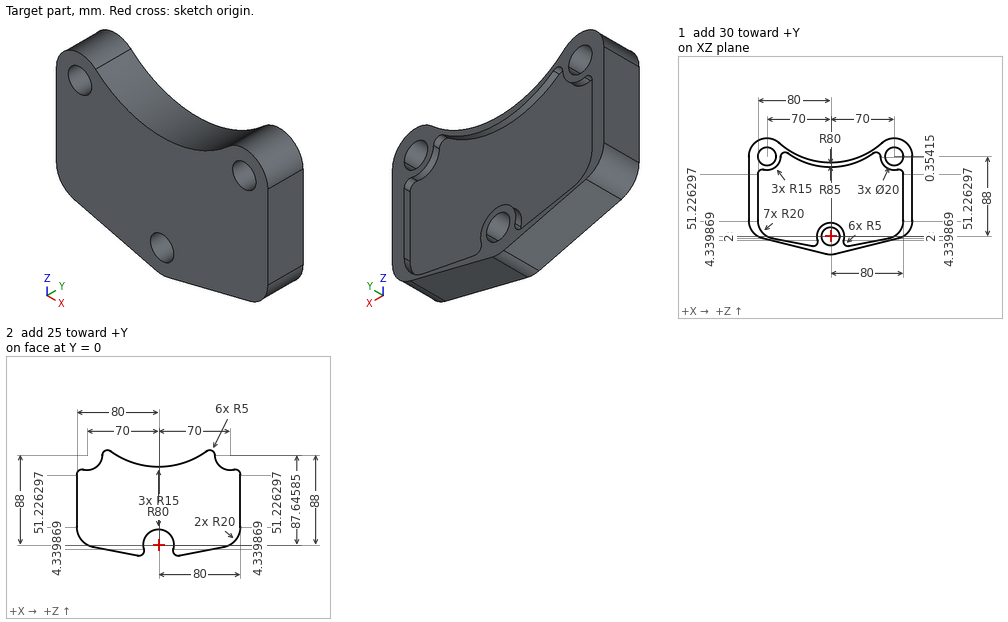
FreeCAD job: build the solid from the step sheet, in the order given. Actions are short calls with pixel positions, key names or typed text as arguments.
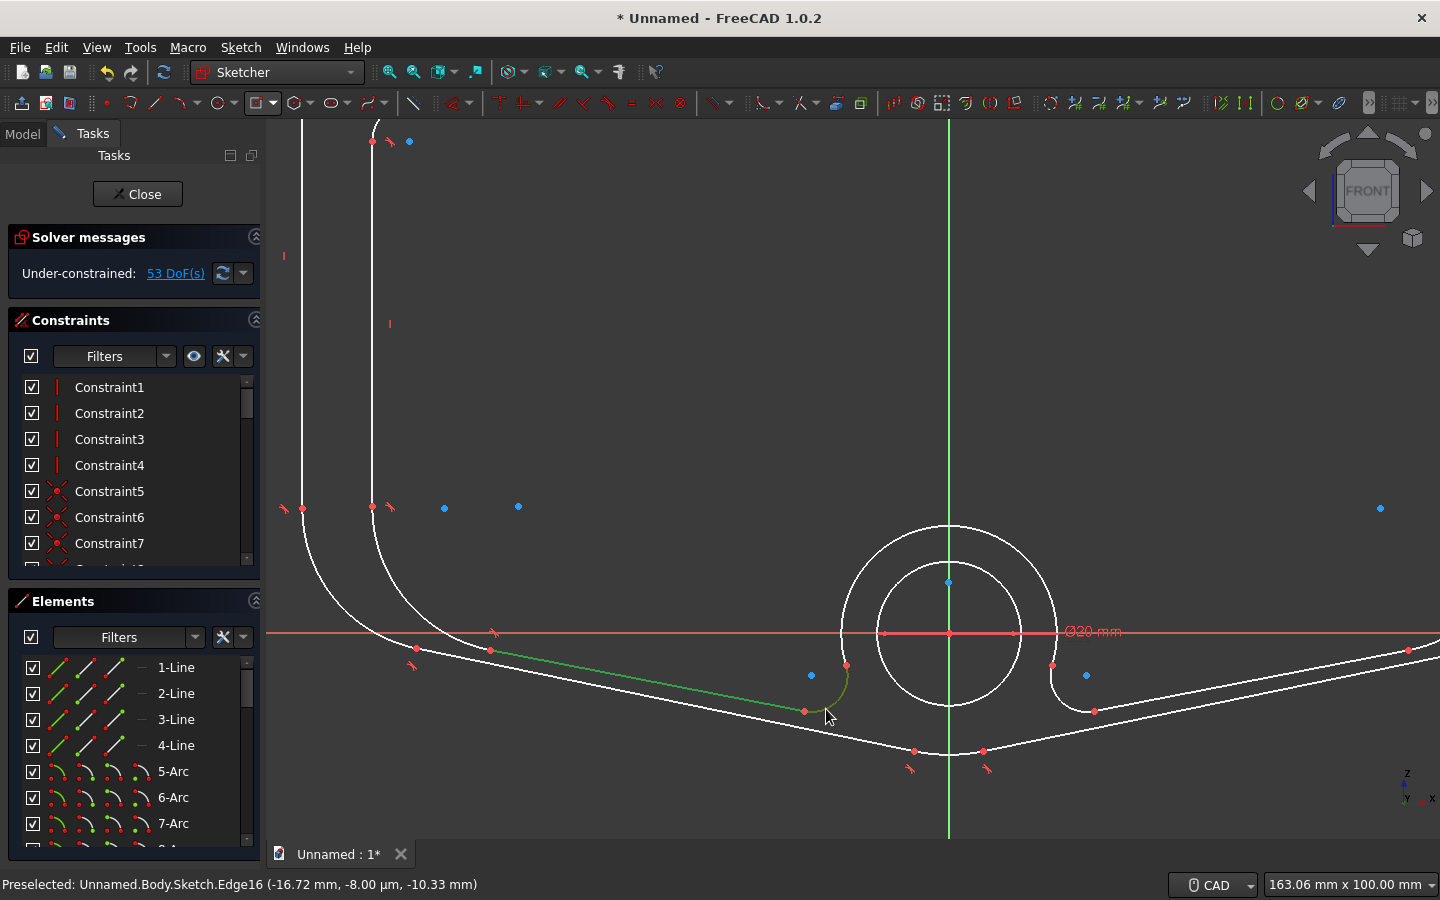
key(t)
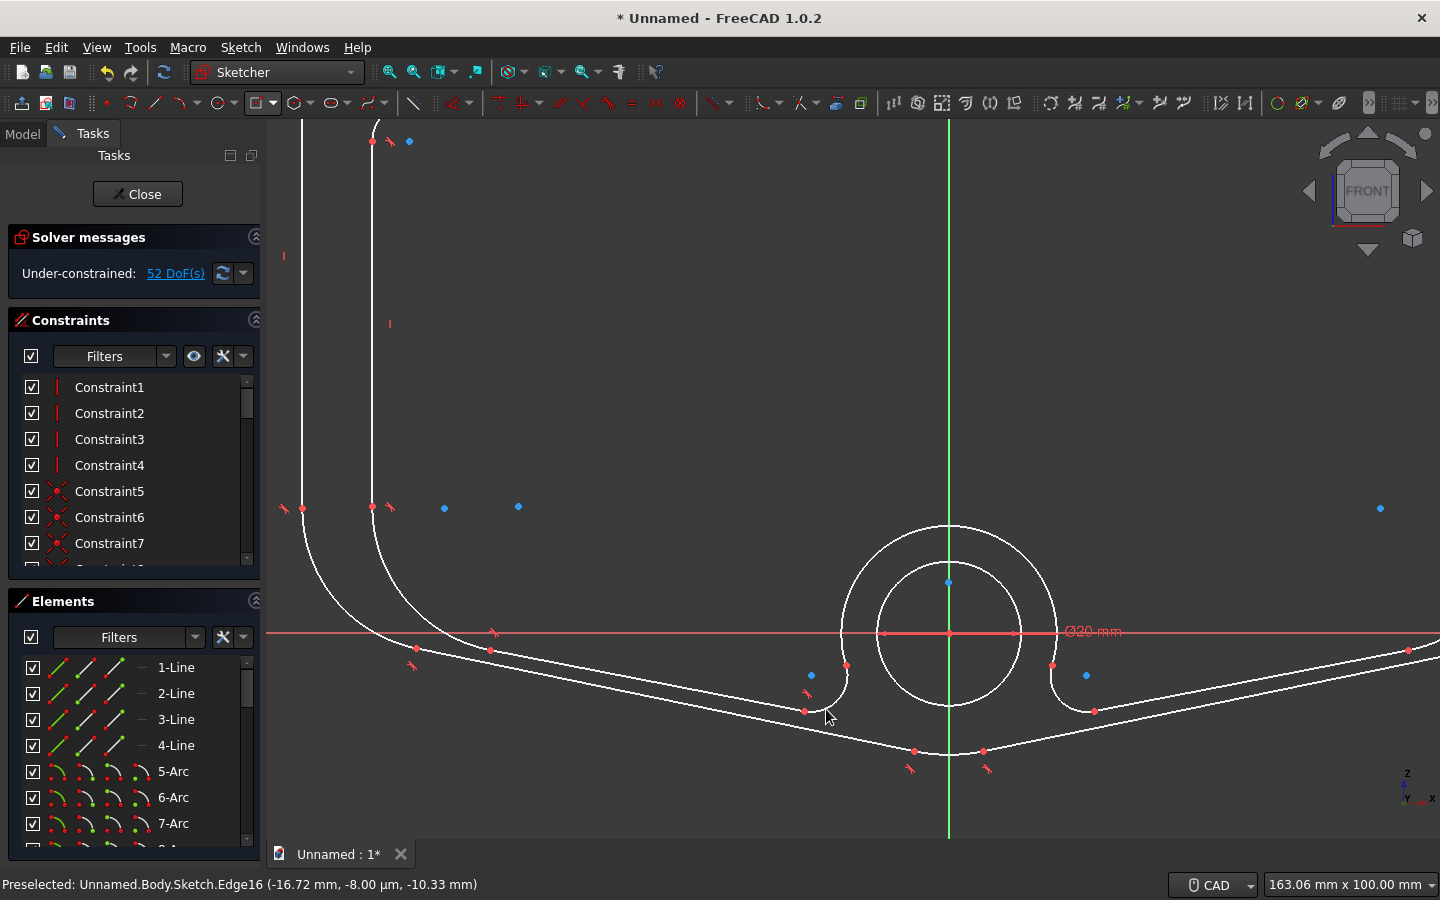
click(1188, 693)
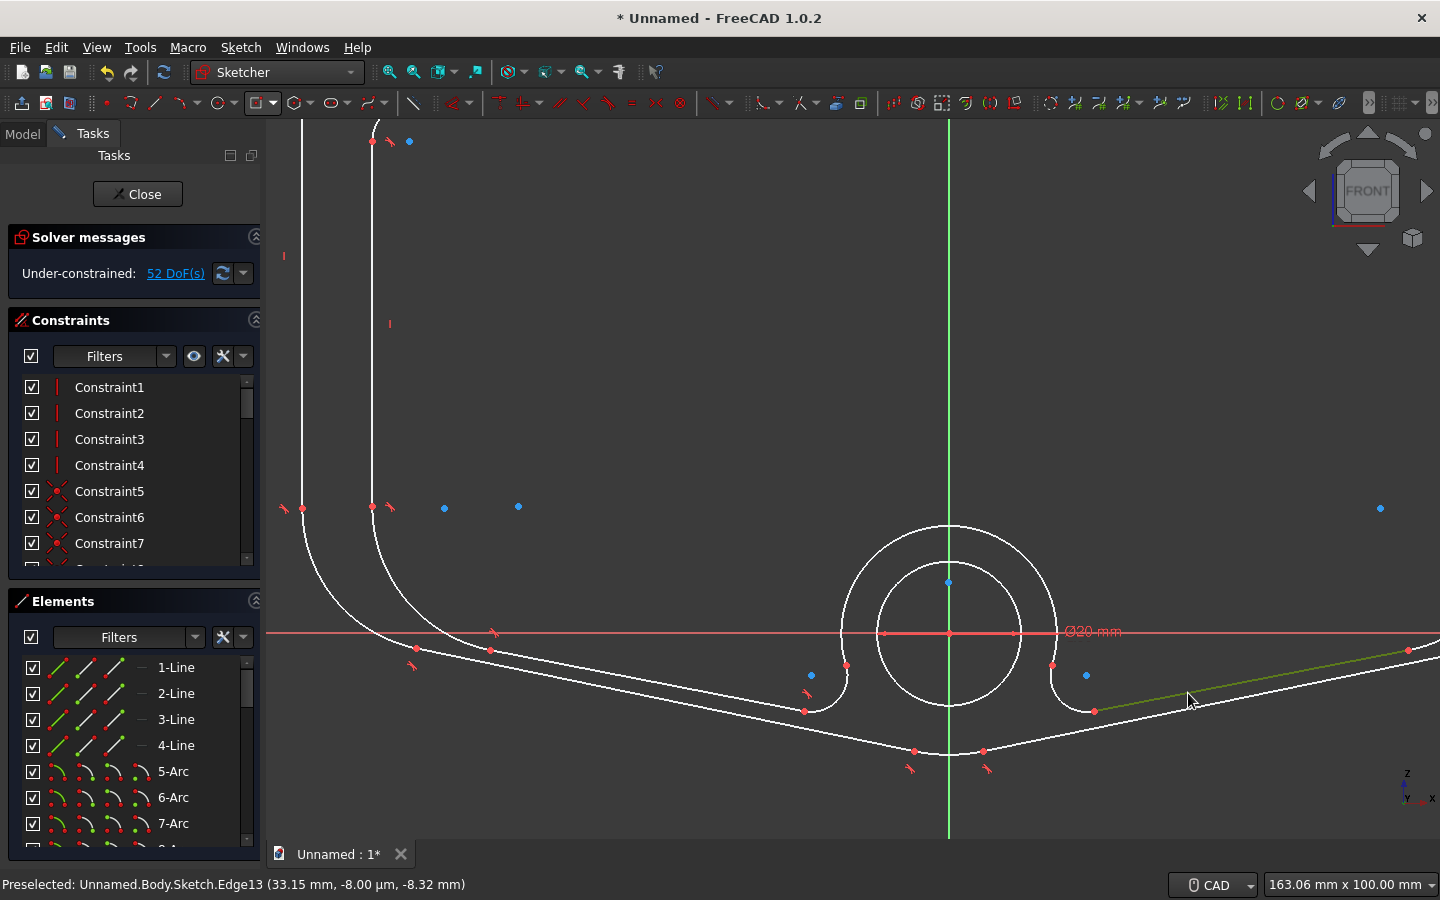
click(1052, 687)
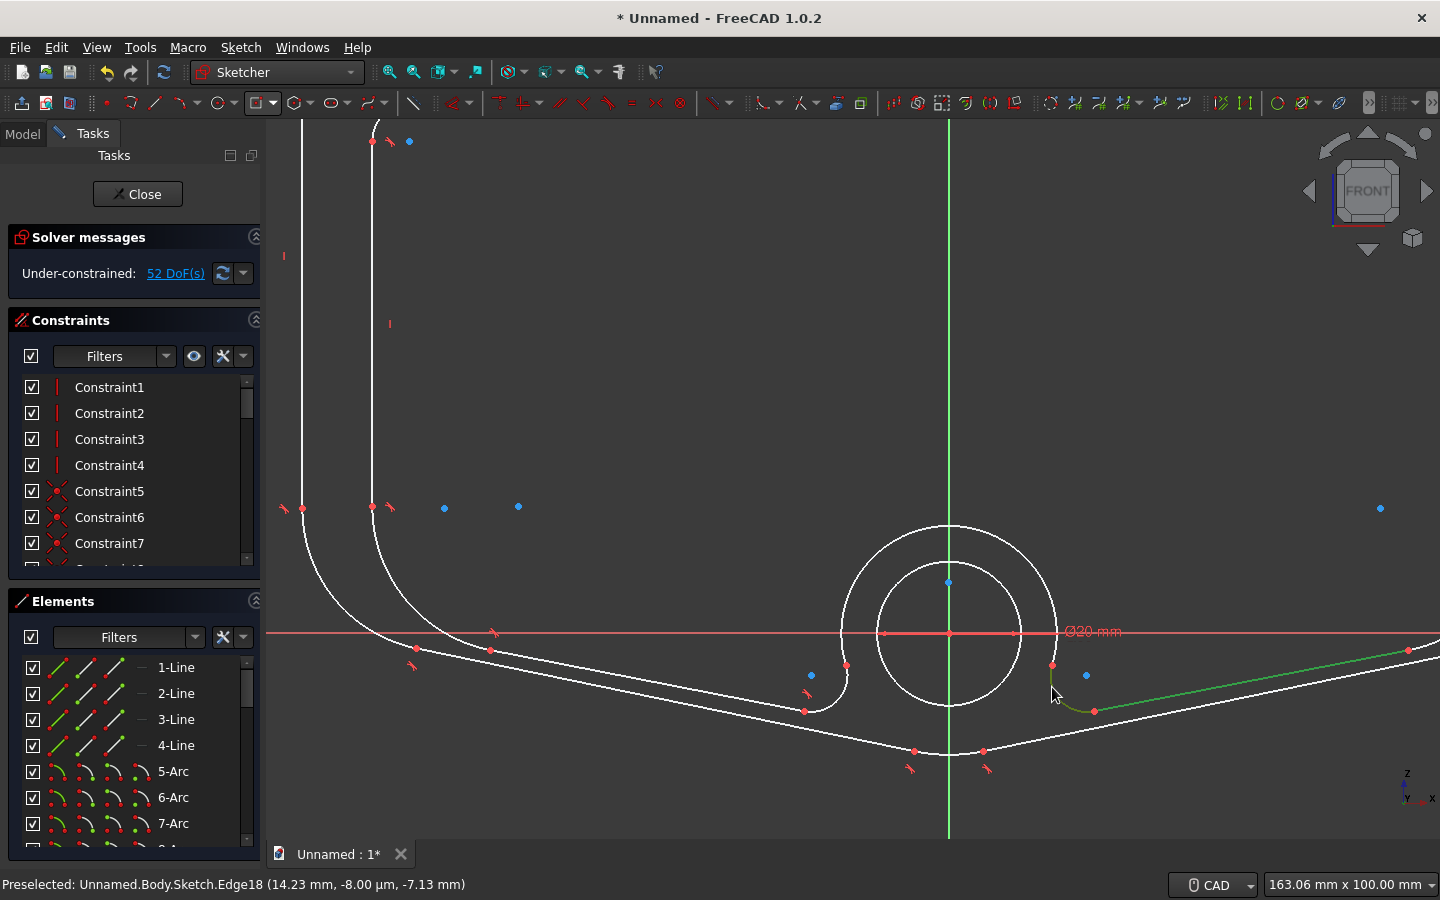
click(608, 104)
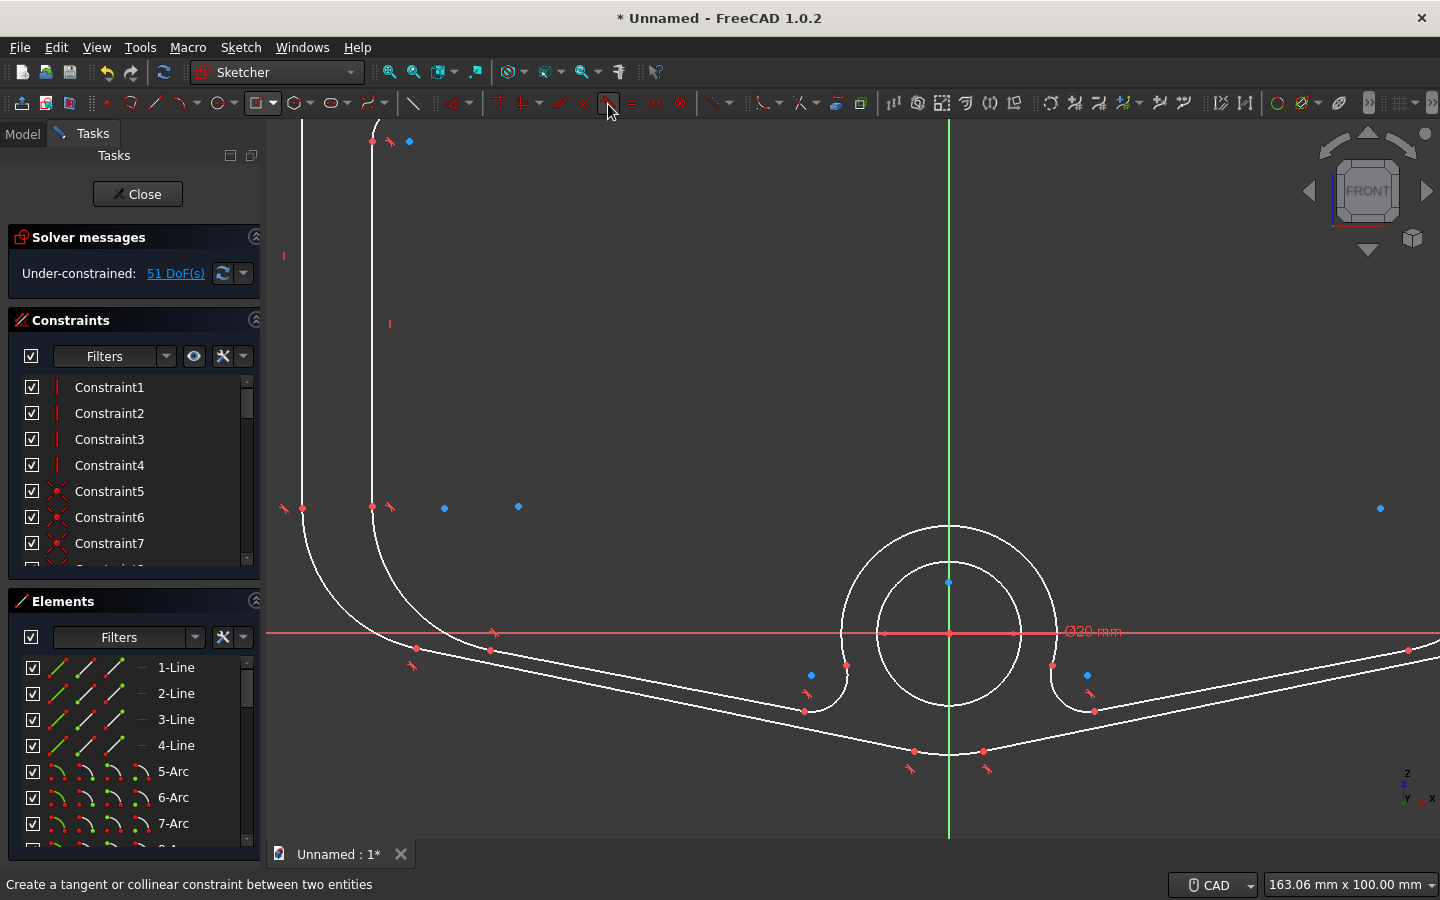
click(1188, 693)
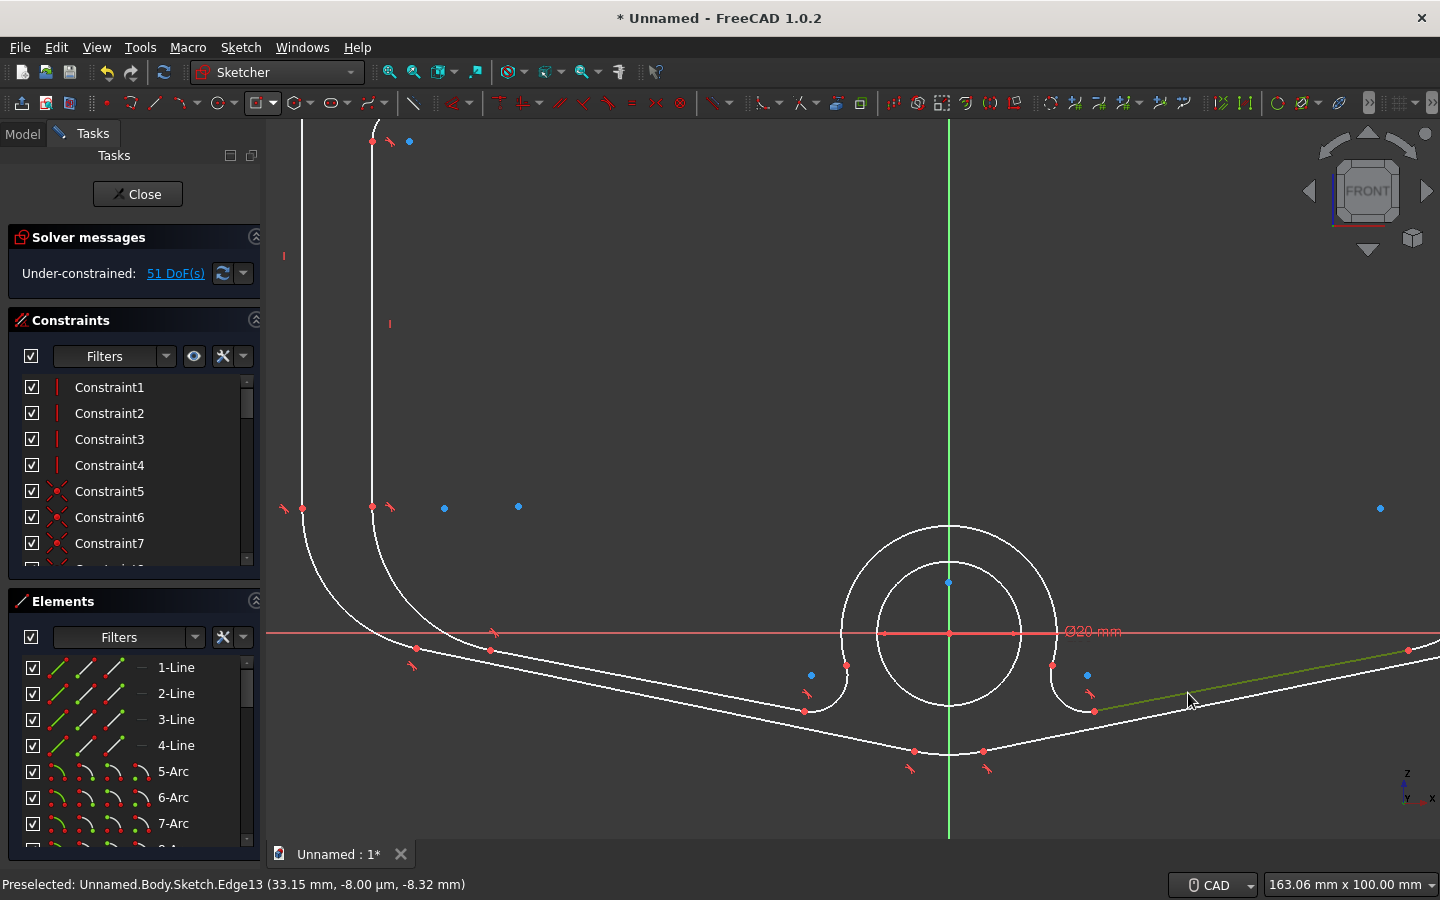
scroll(584, 669, down, 3)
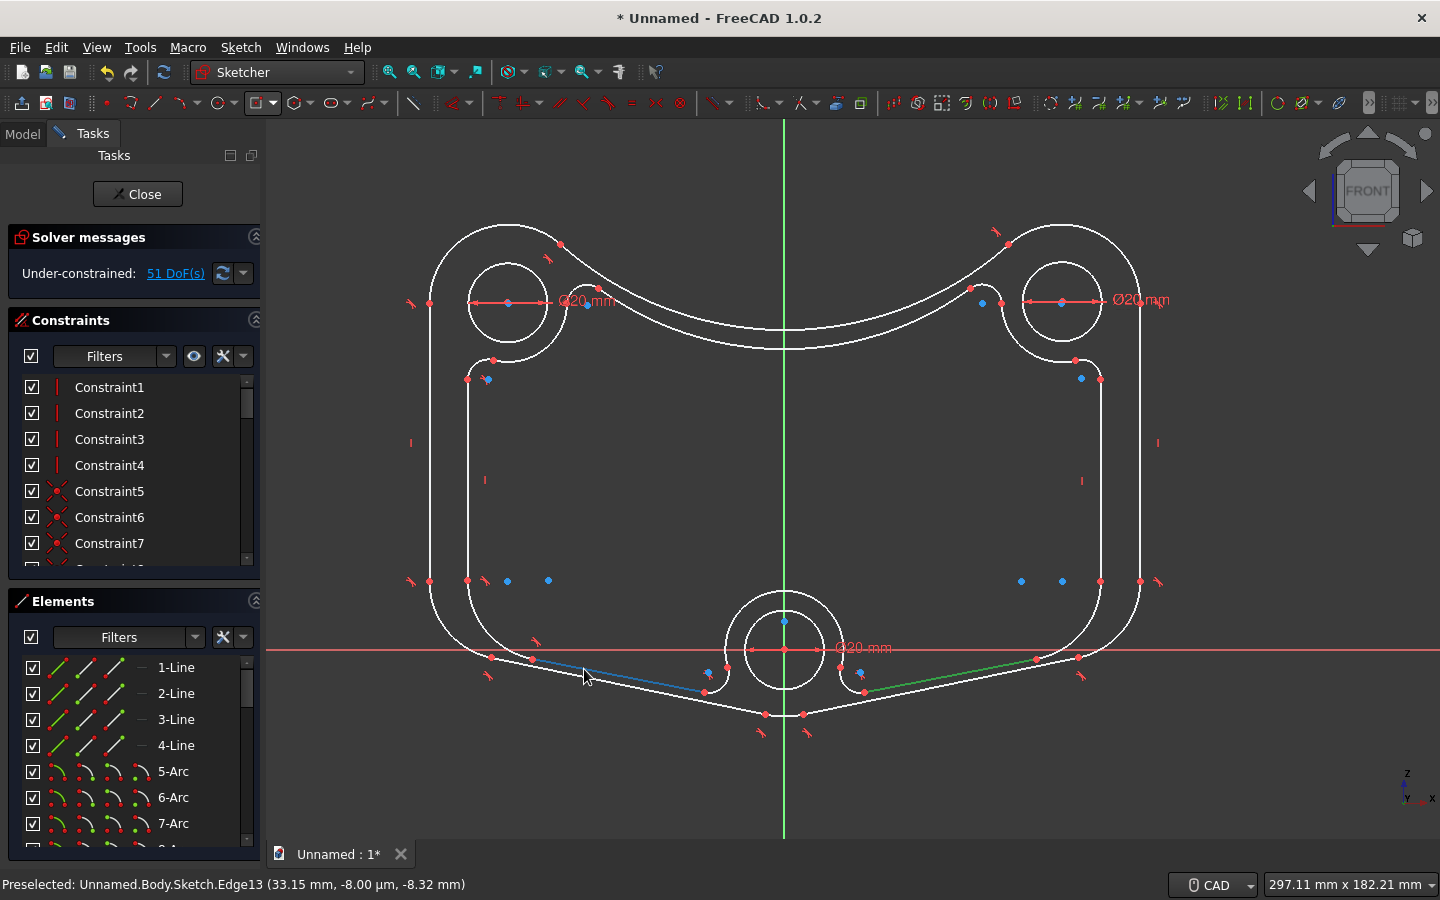
click(1094, 613)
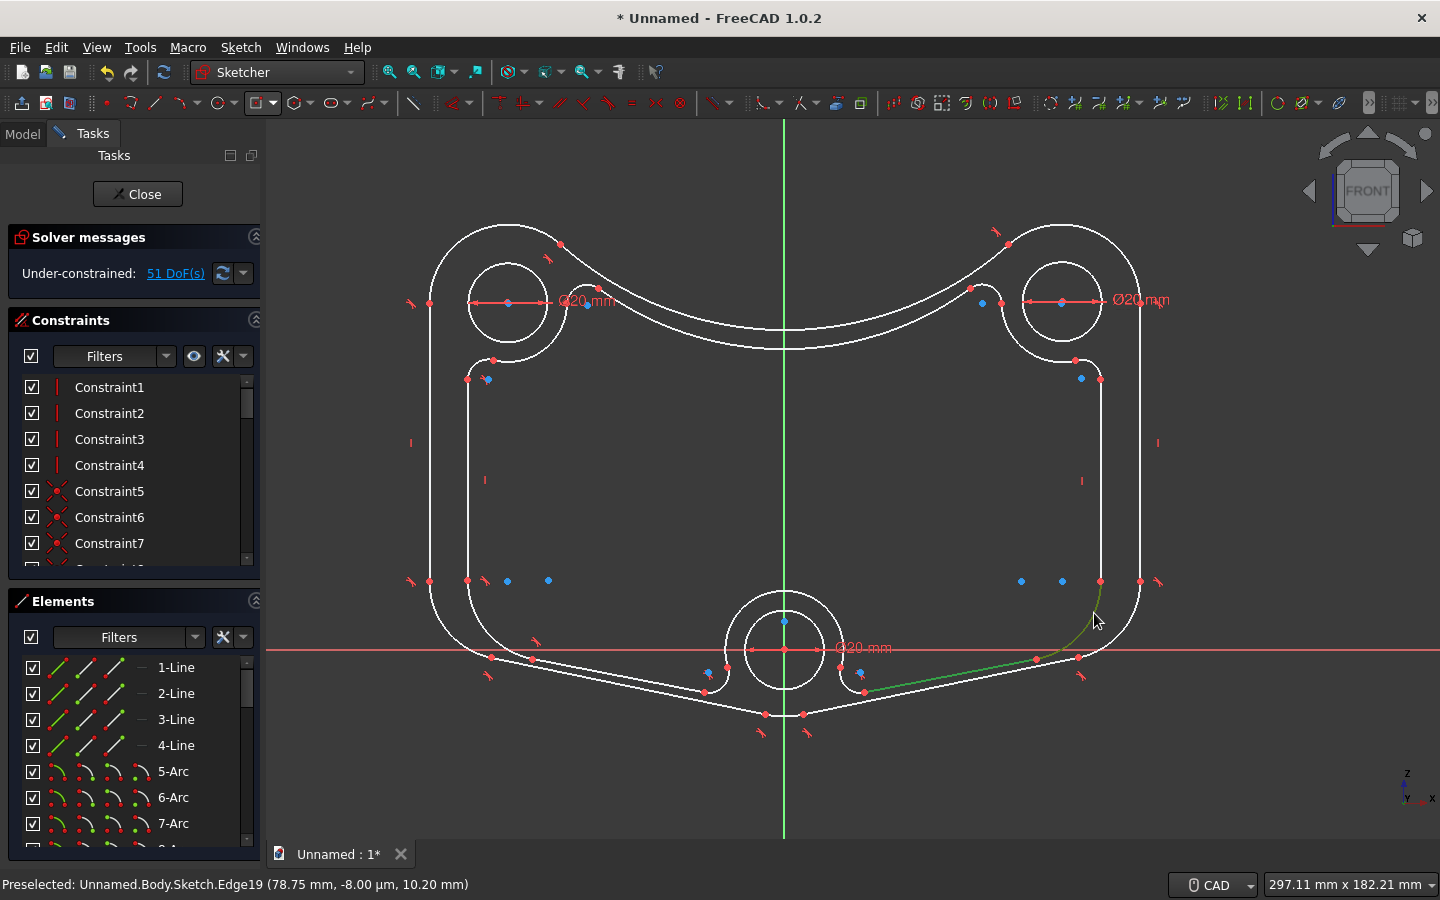
click(608, 104)